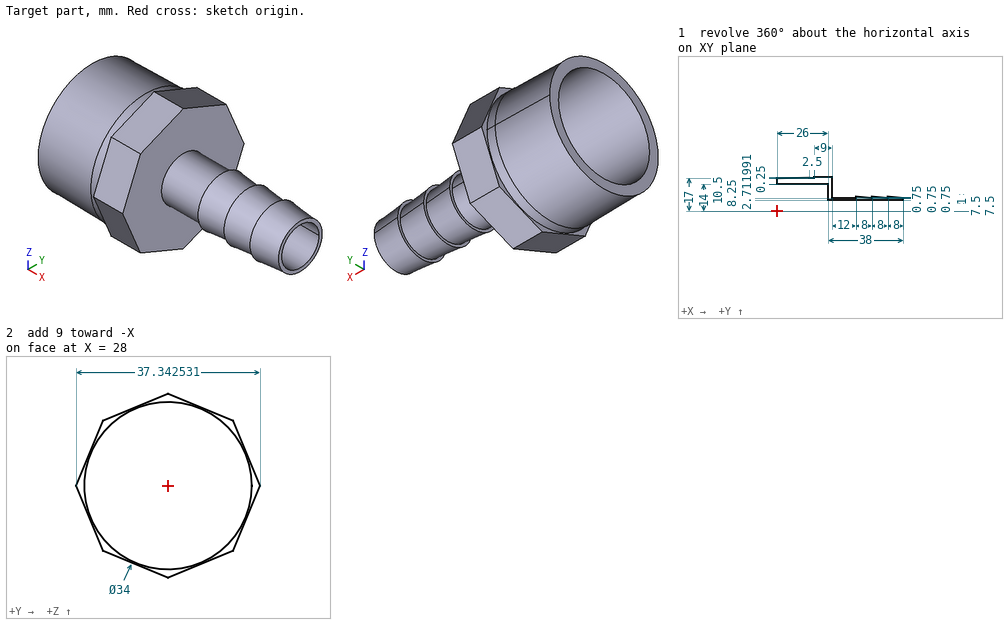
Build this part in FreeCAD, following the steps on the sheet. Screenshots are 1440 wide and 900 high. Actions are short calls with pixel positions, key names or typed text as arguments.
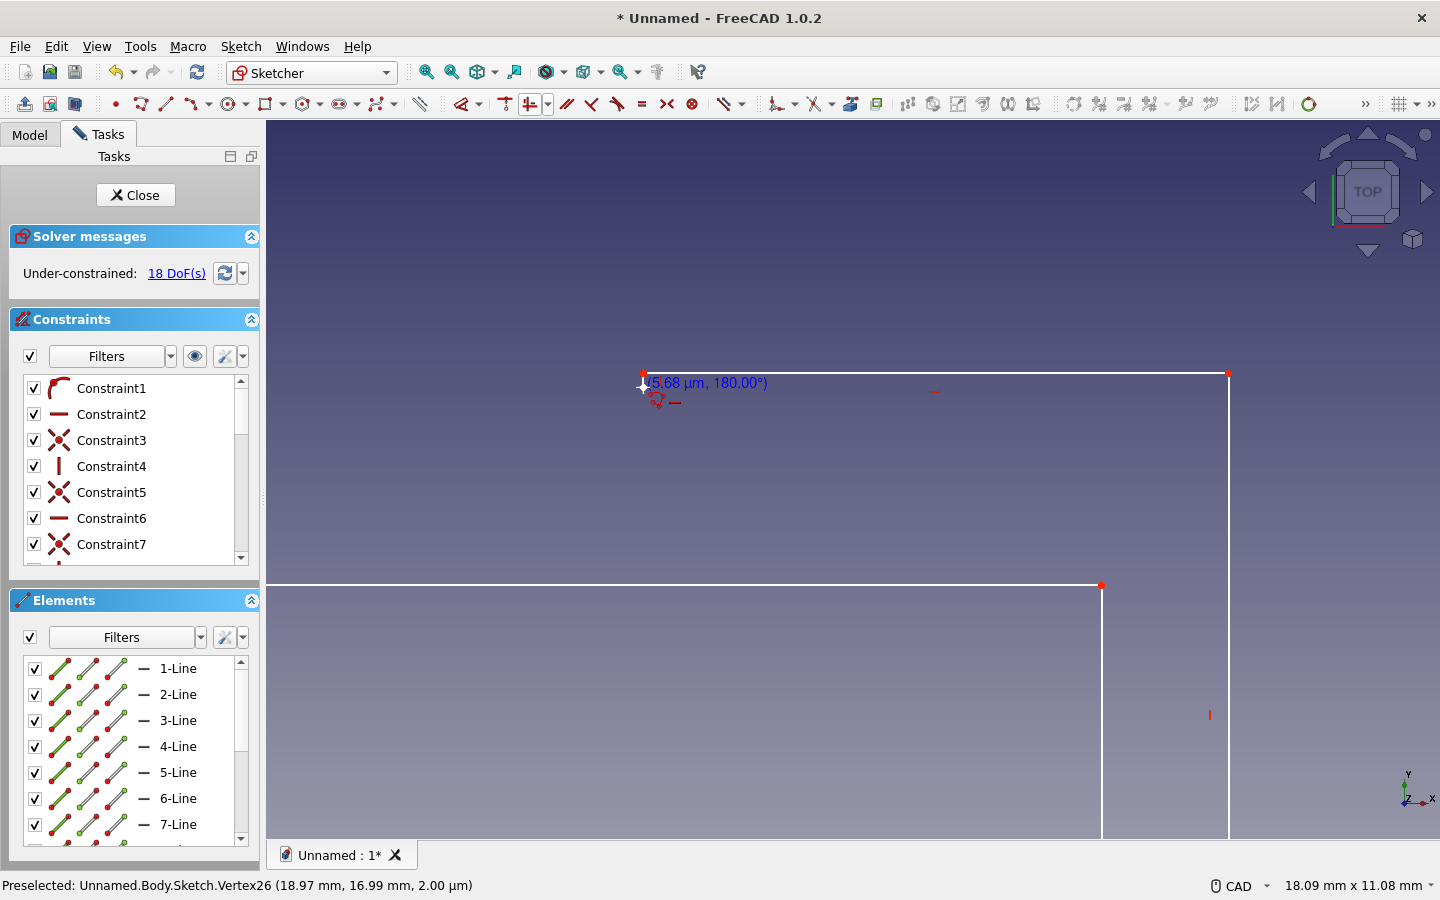
scroll(645, 390, down, 9)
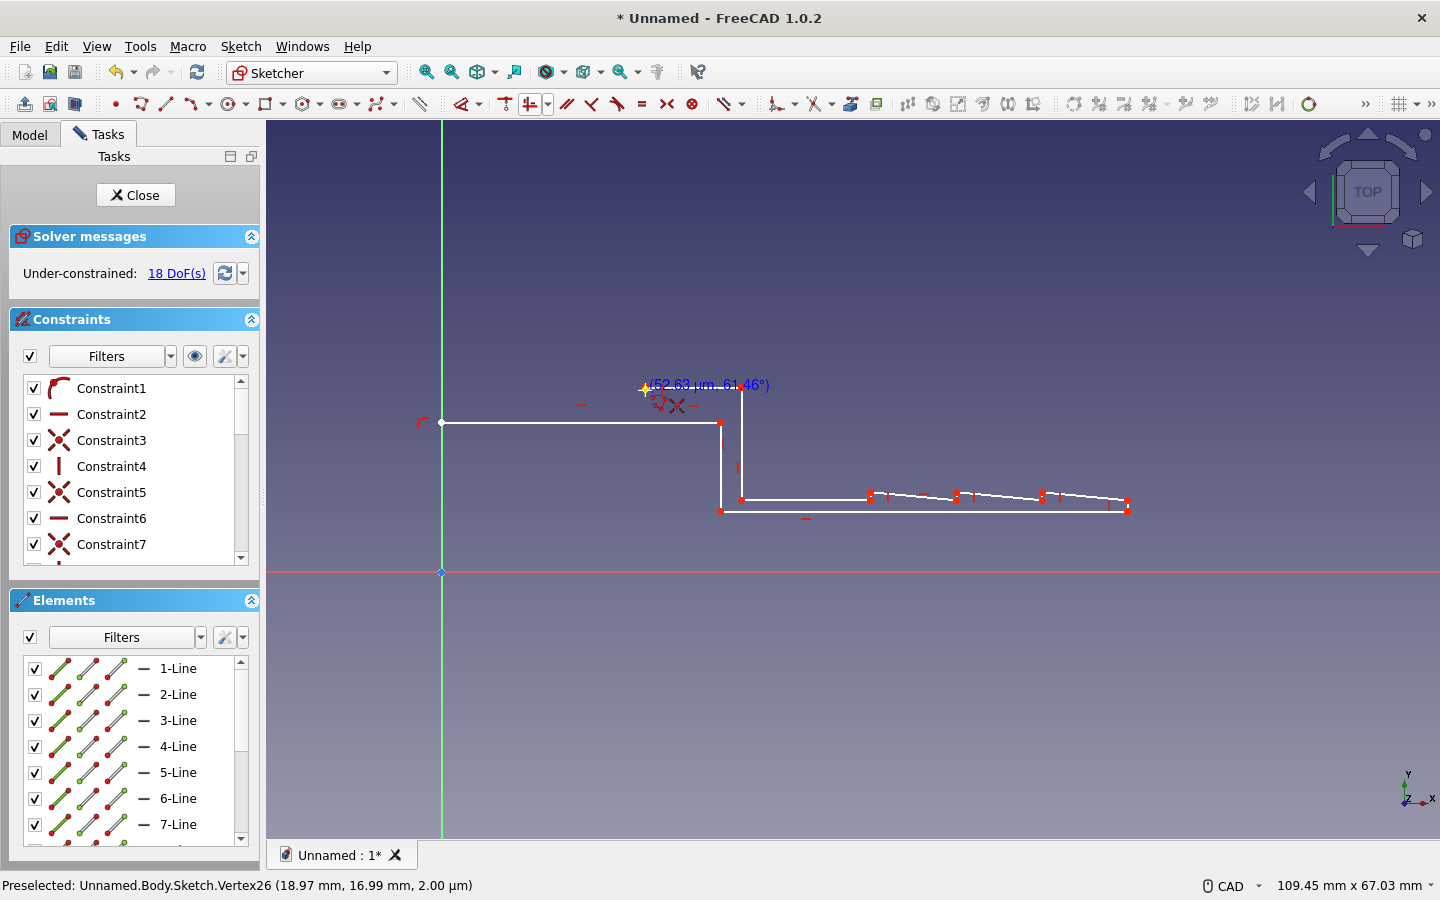
click(619, 390)
click(451, 399)
click(442, 423)
key(Escape)
key(Escape)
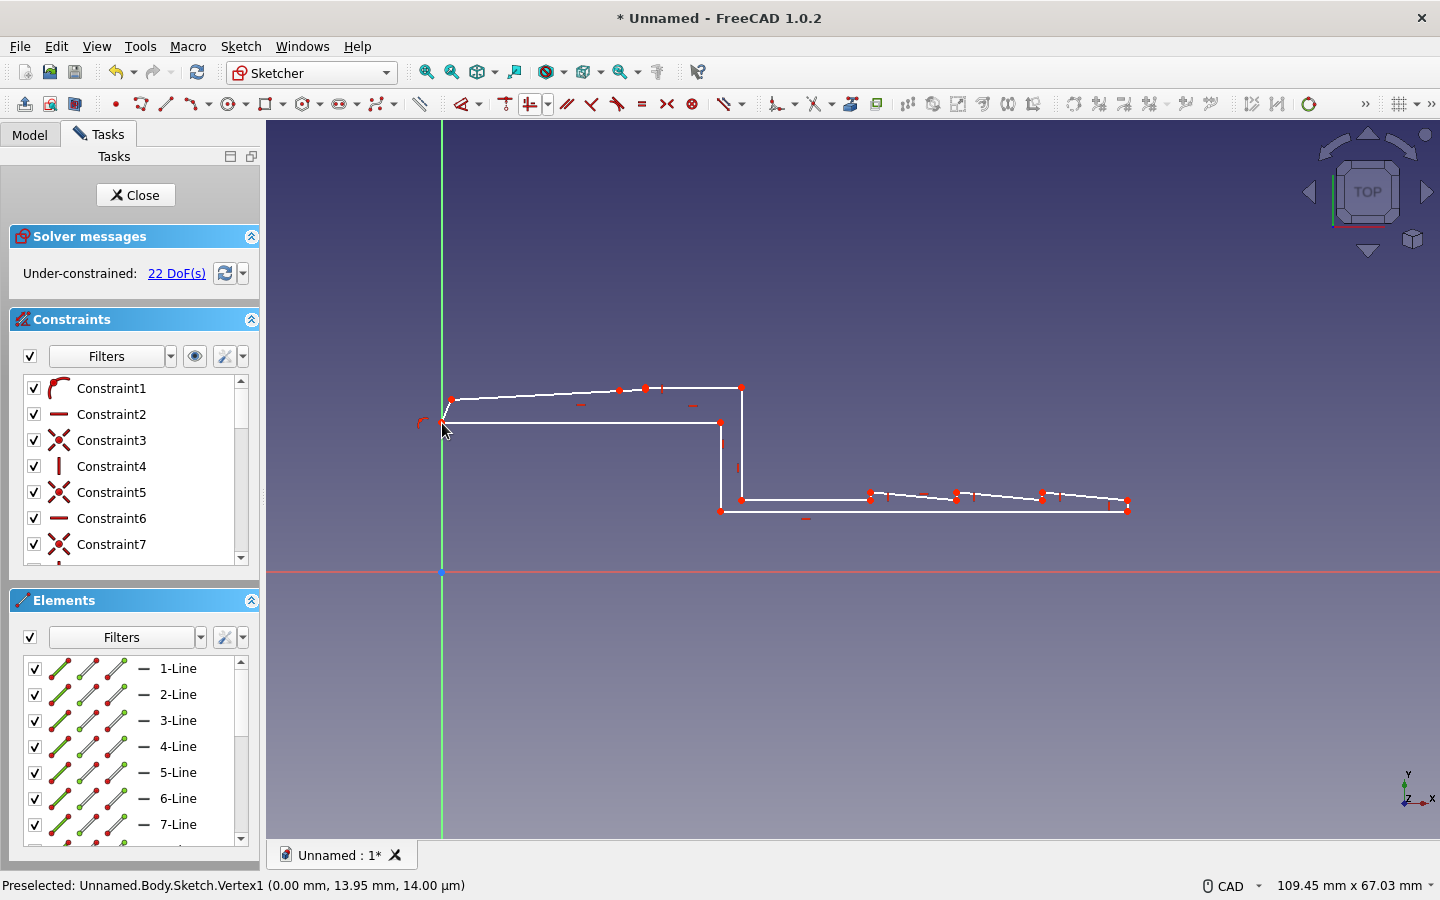
scroll(635, 390, up, 2)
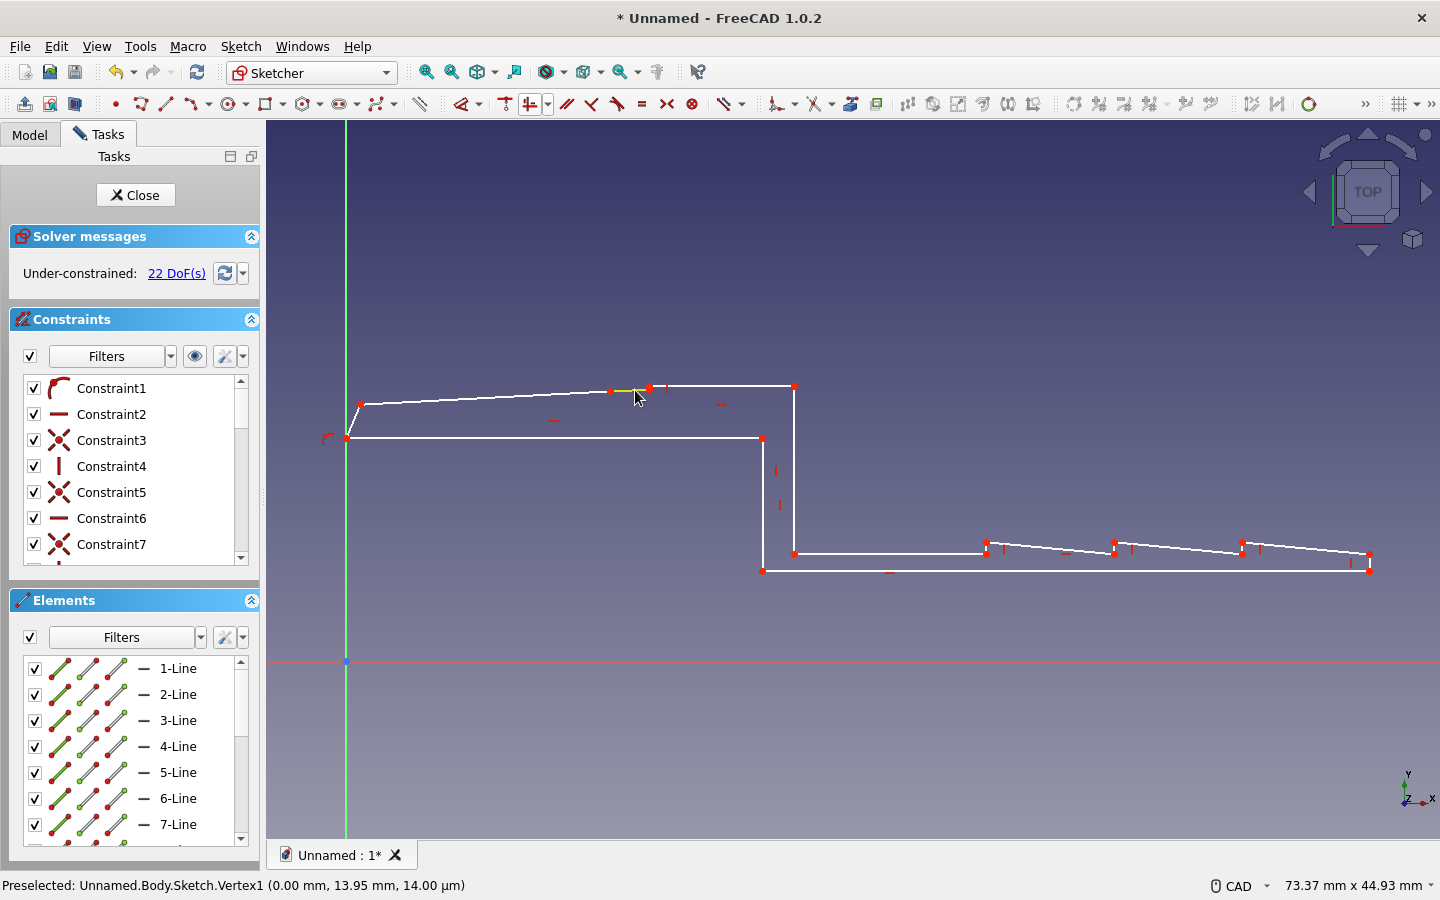
click(634, 390)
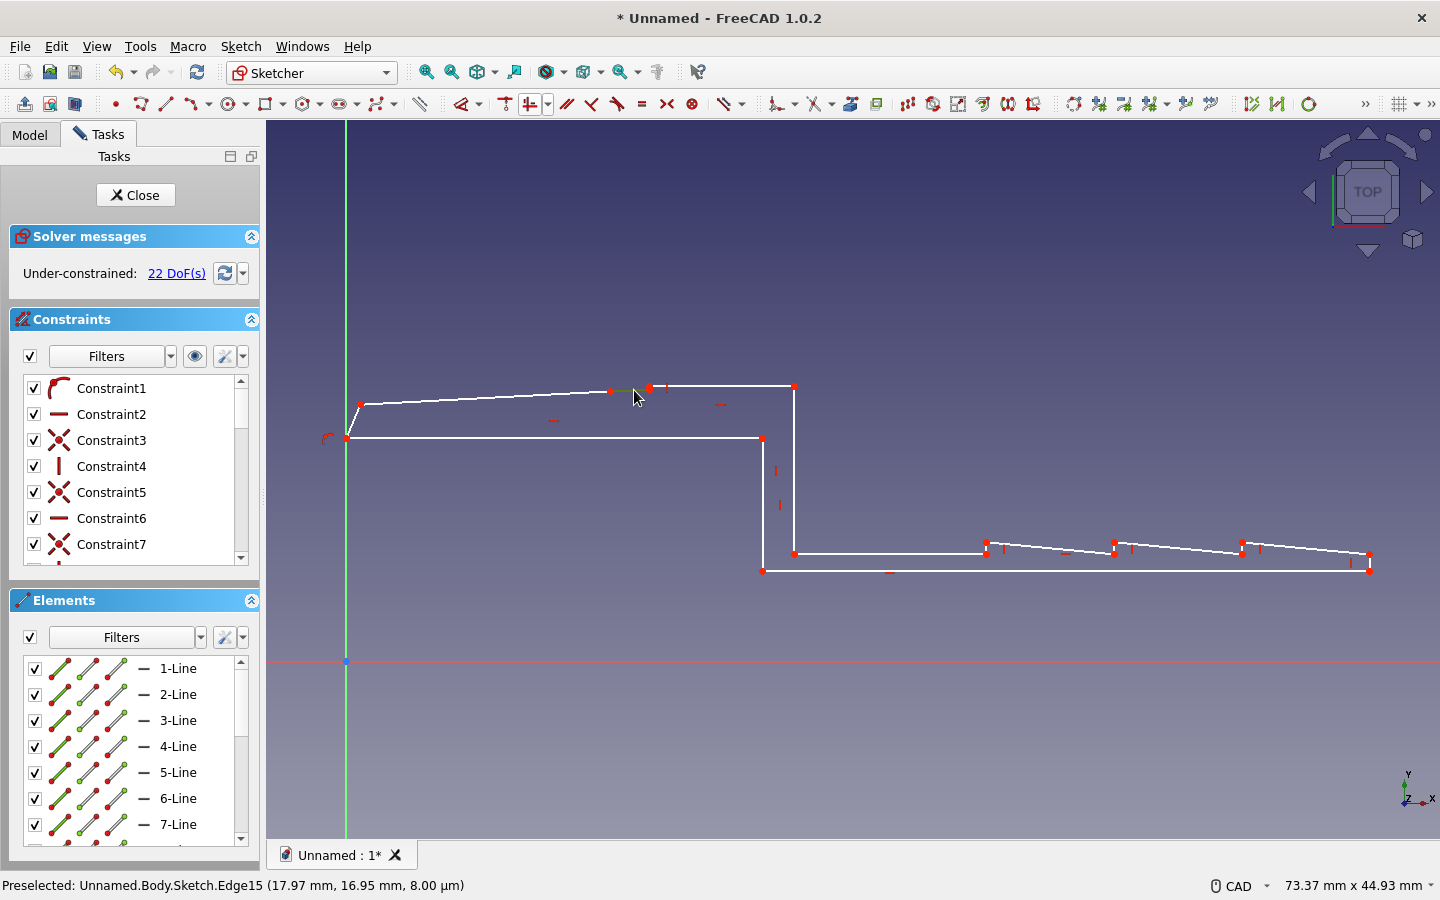
key(h)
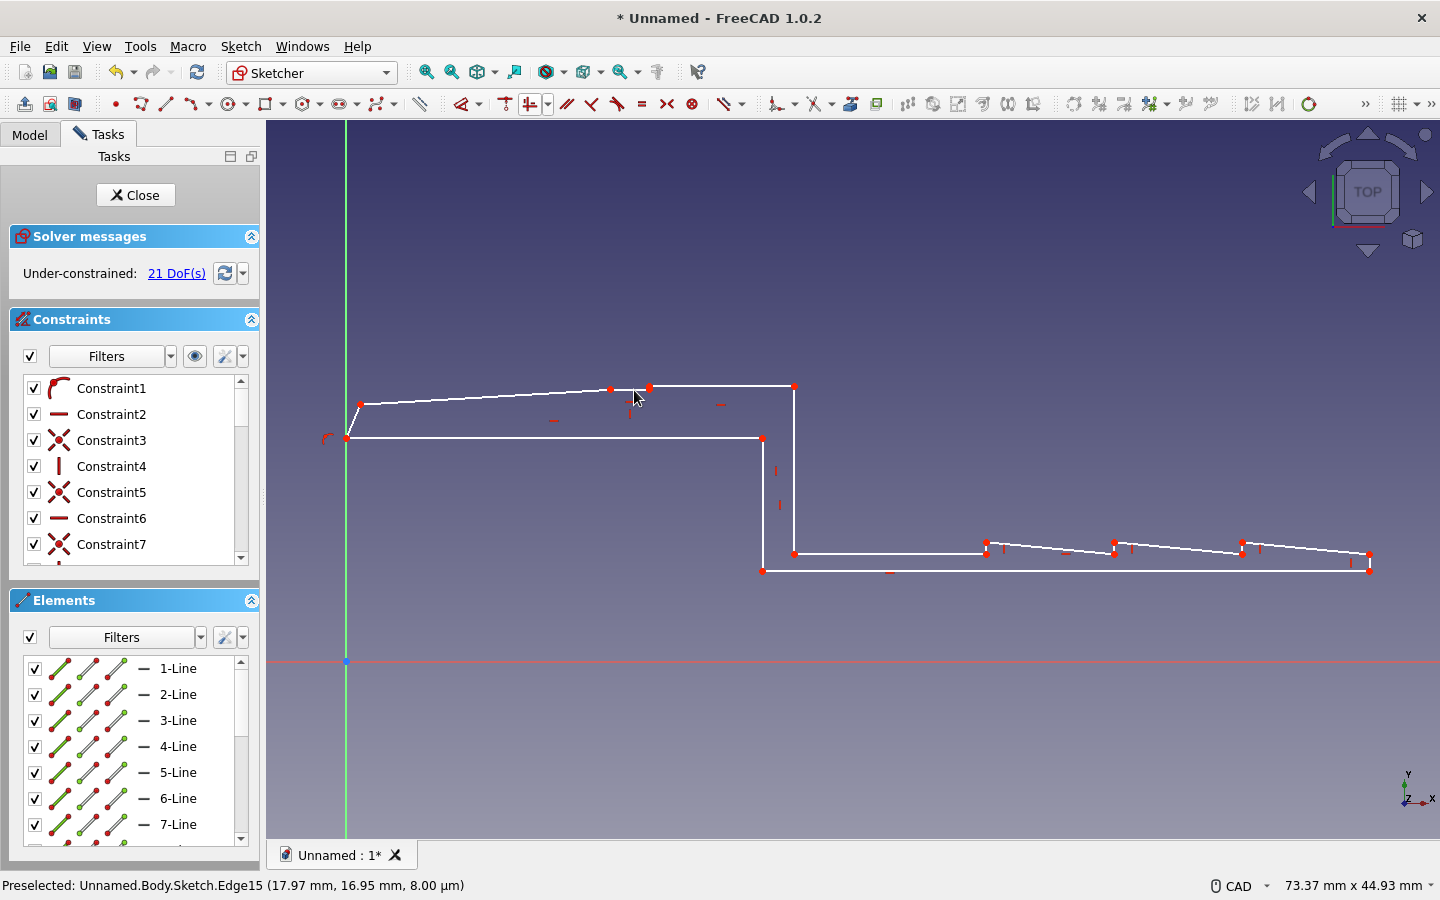
scroll(356, 415, up, 2)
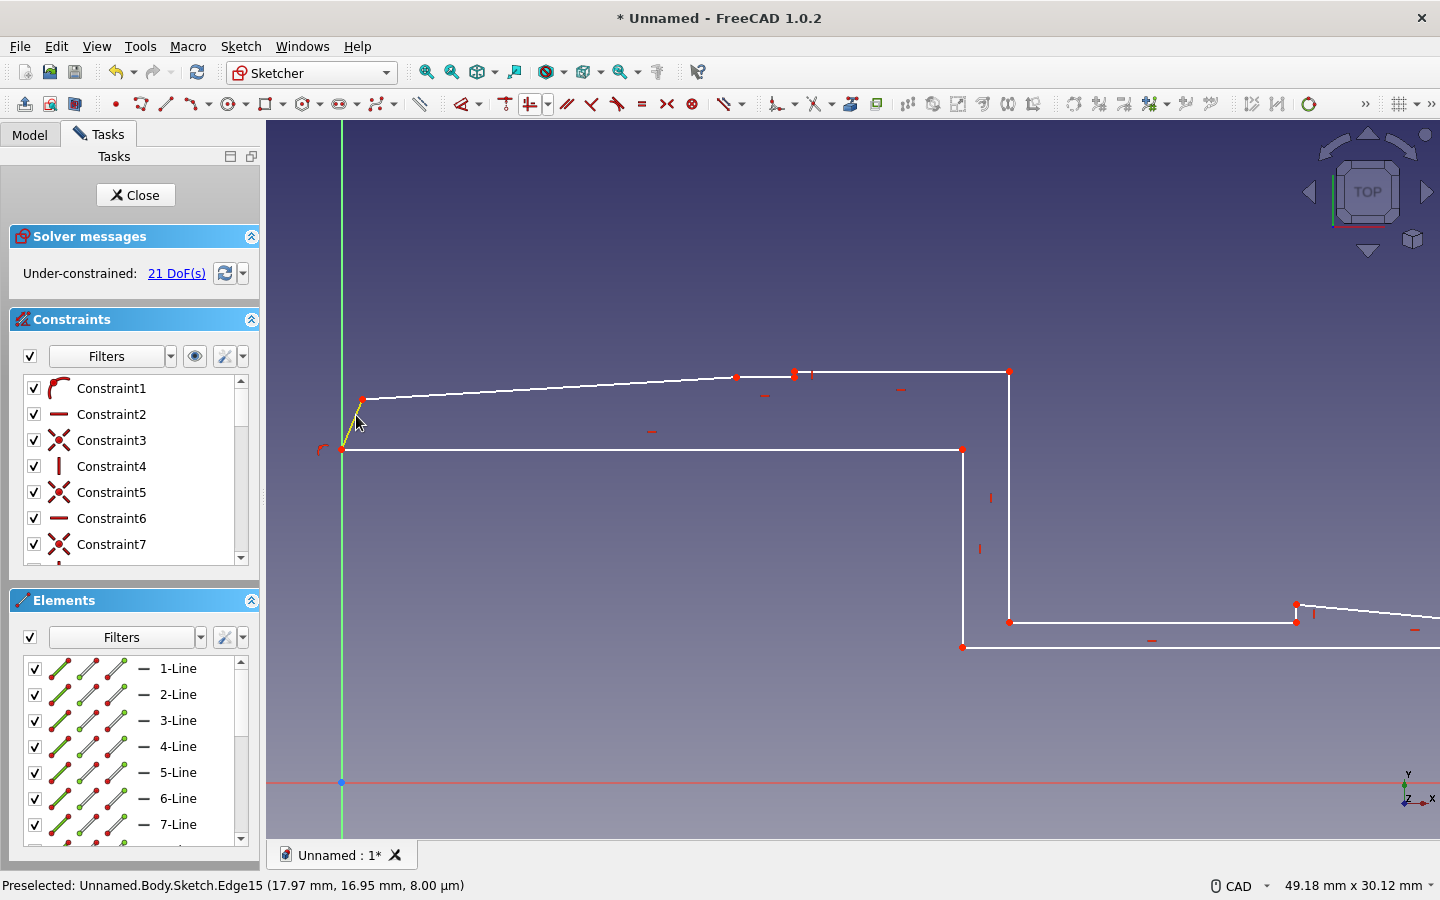
click(356, 415)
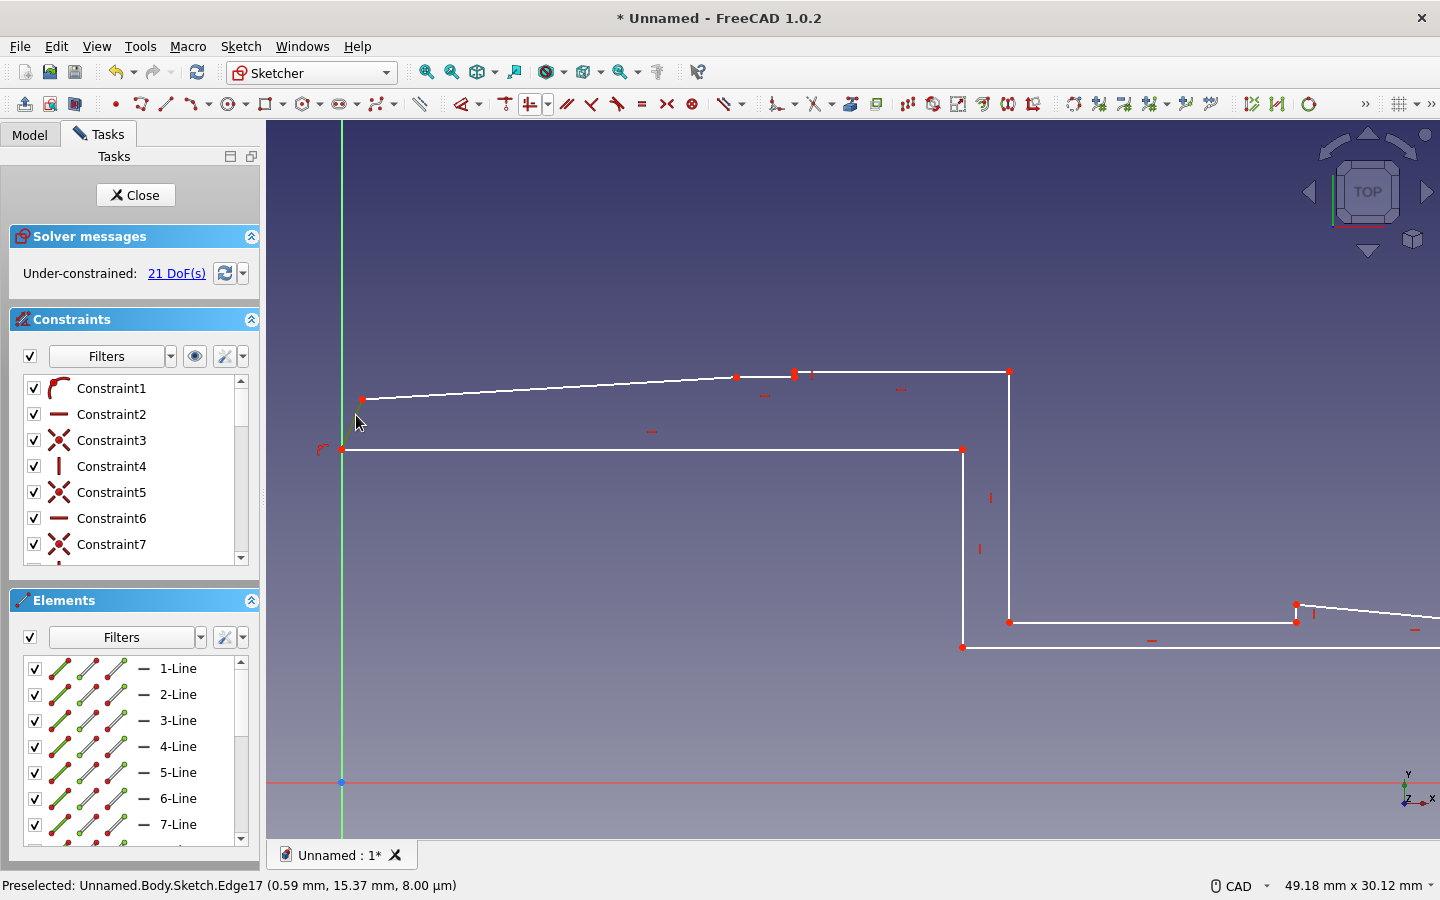
click(548, 104)